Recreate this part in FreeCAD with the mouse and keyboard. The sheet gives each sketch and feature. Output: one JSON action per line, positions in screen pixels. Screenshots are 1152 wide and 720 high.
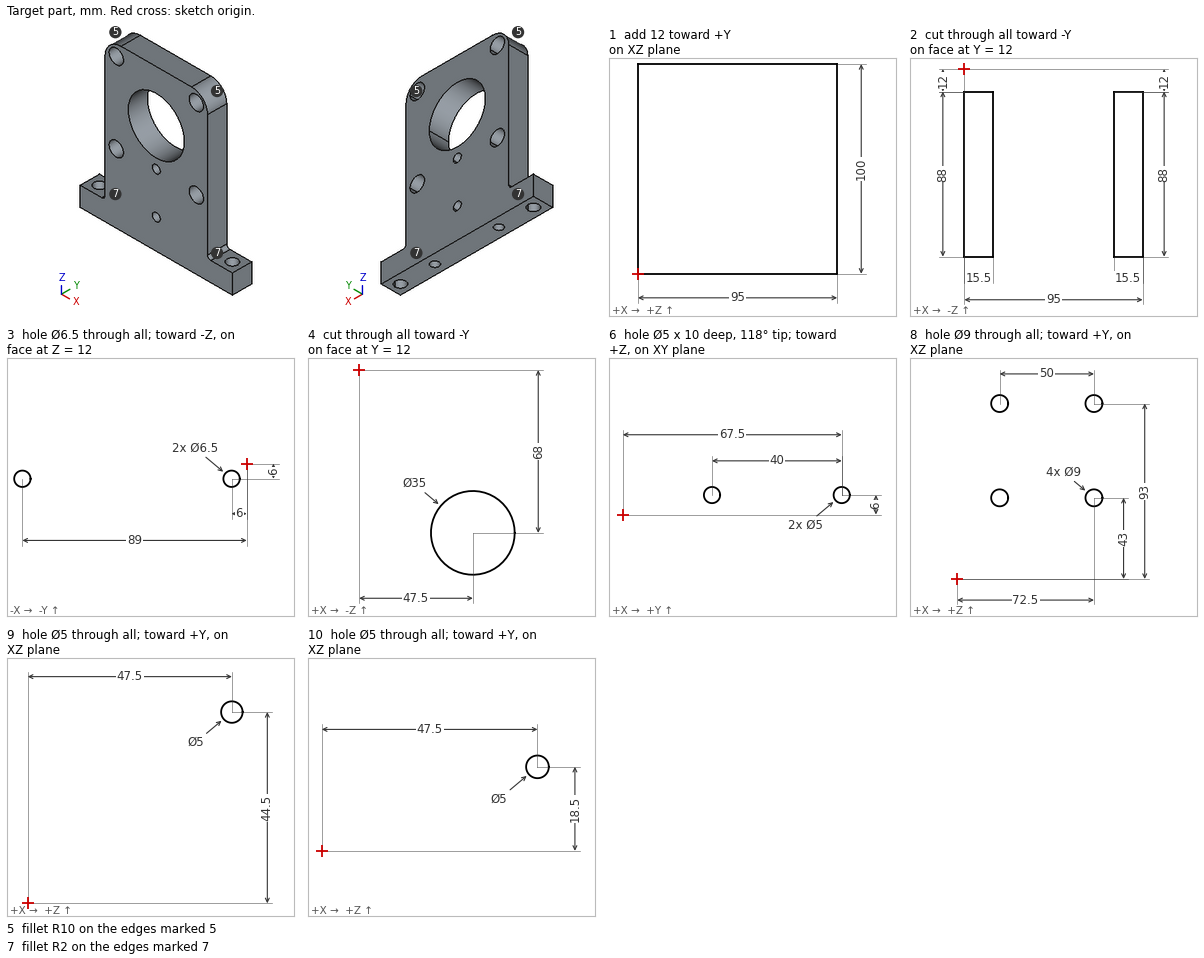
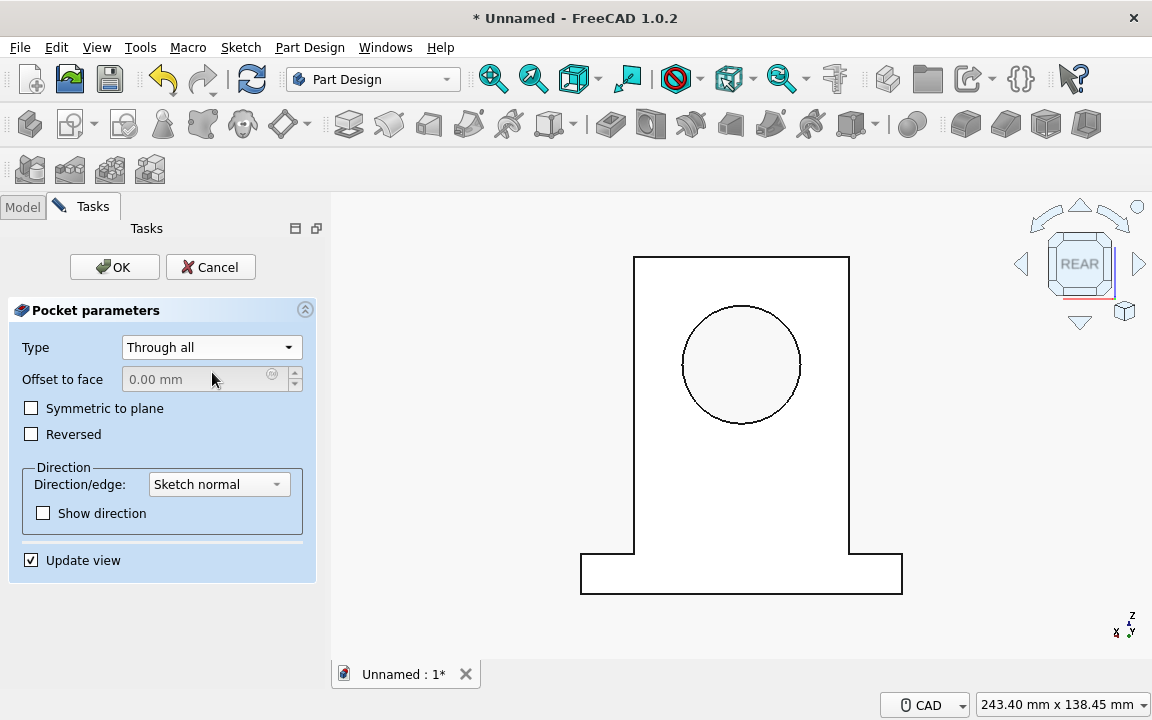
{"action": "left_click", "coordinate": [115, 267]}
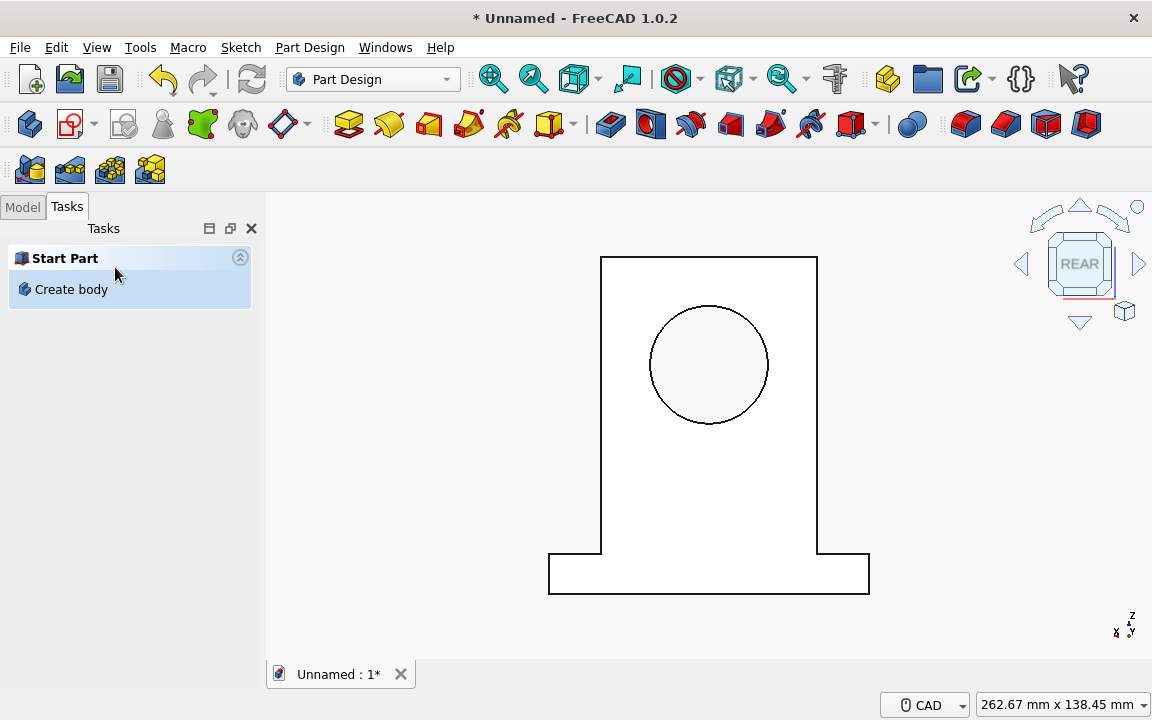
{"action": "key", "text": "0"}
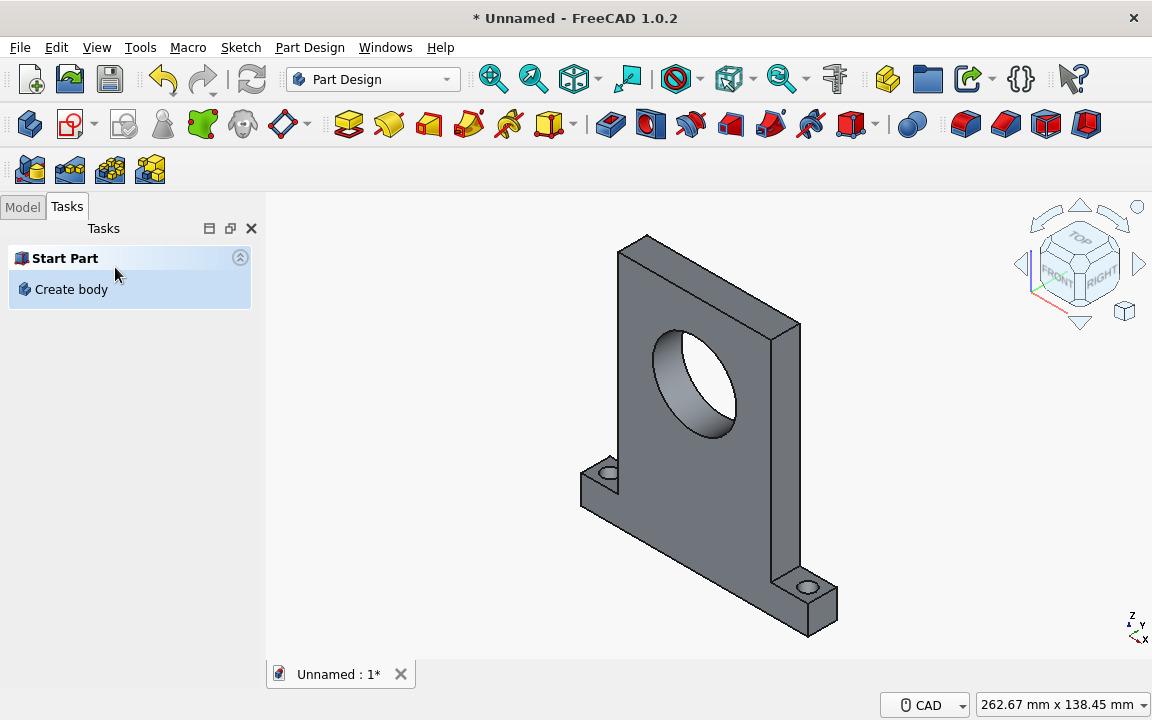
{"action": "left_click", "coordinate": [785, 331]}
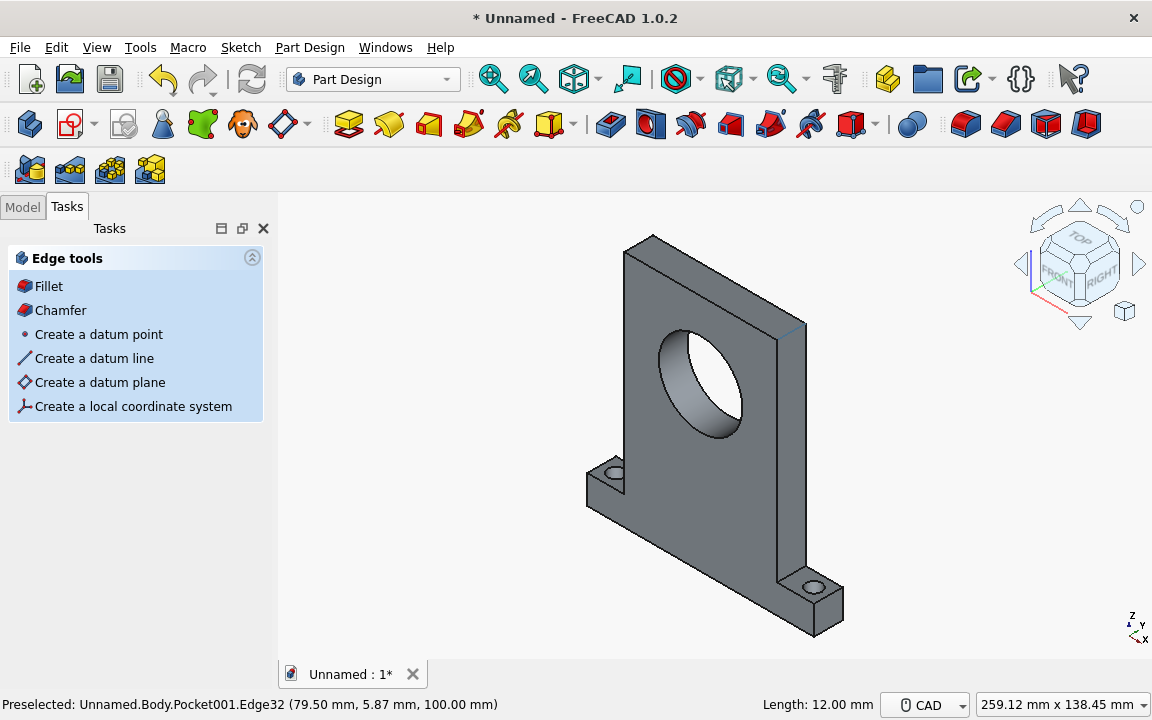
{"action": "key", "text": "2"}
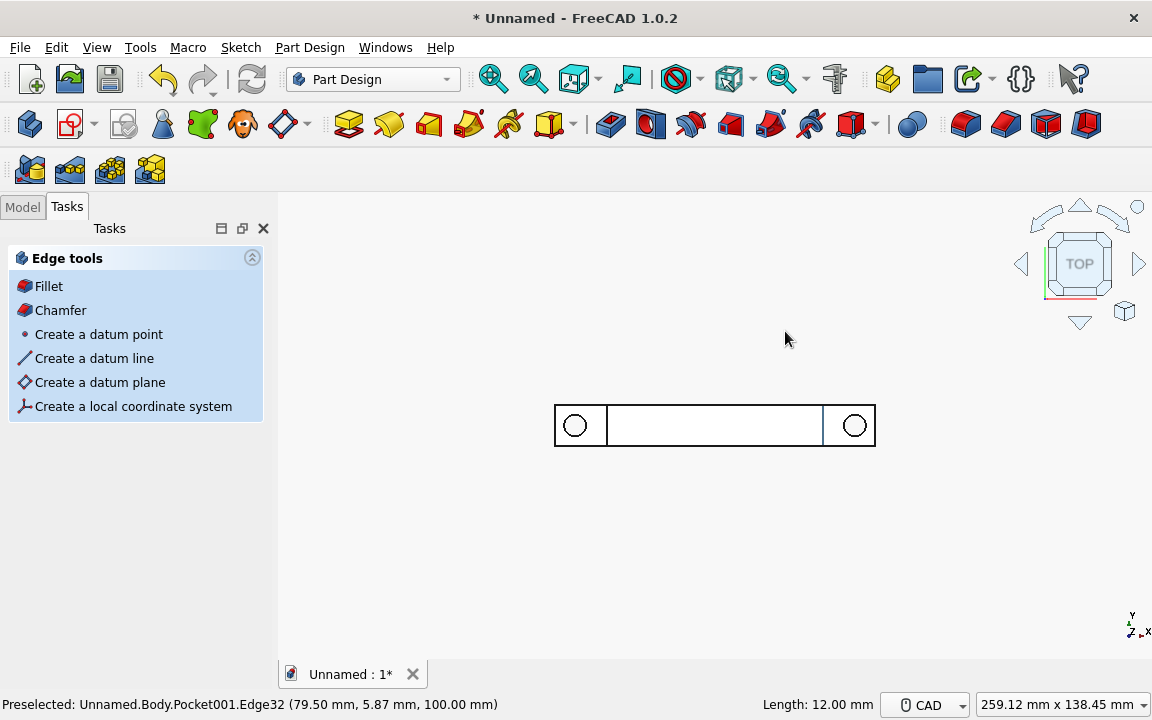
{"action": "left_click", "coordinate": [494, 80]}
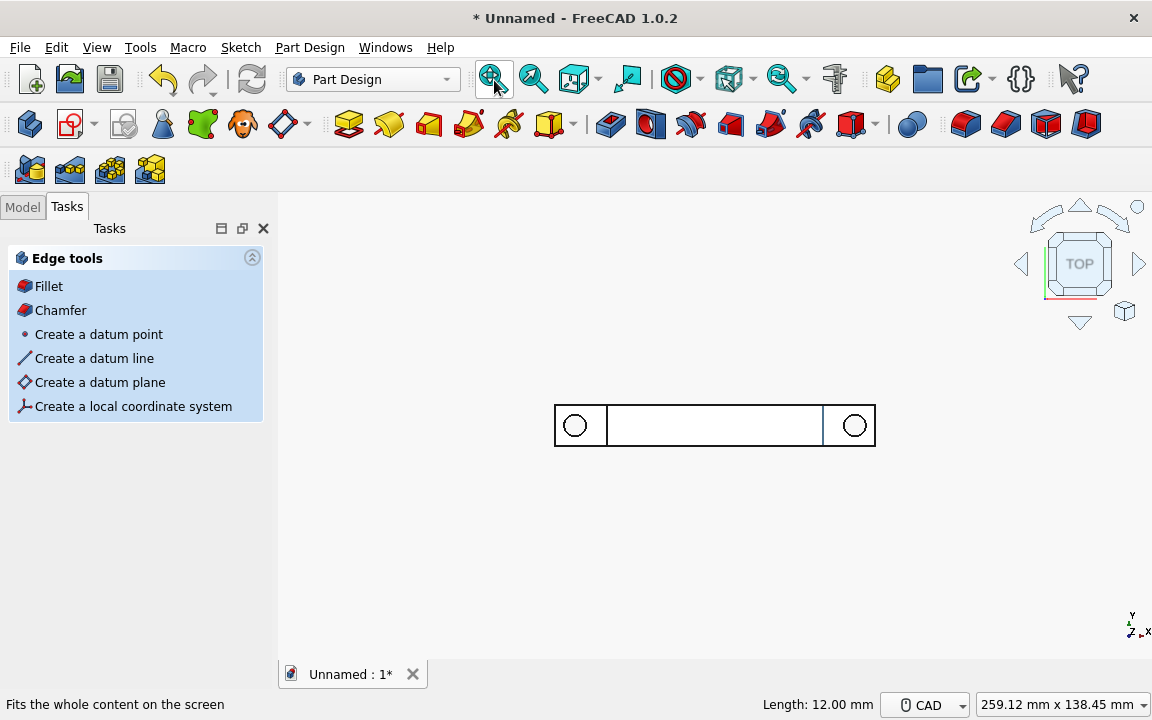
{"action": "left_click", "coordinate": [607, 424], "text": "ctrl"}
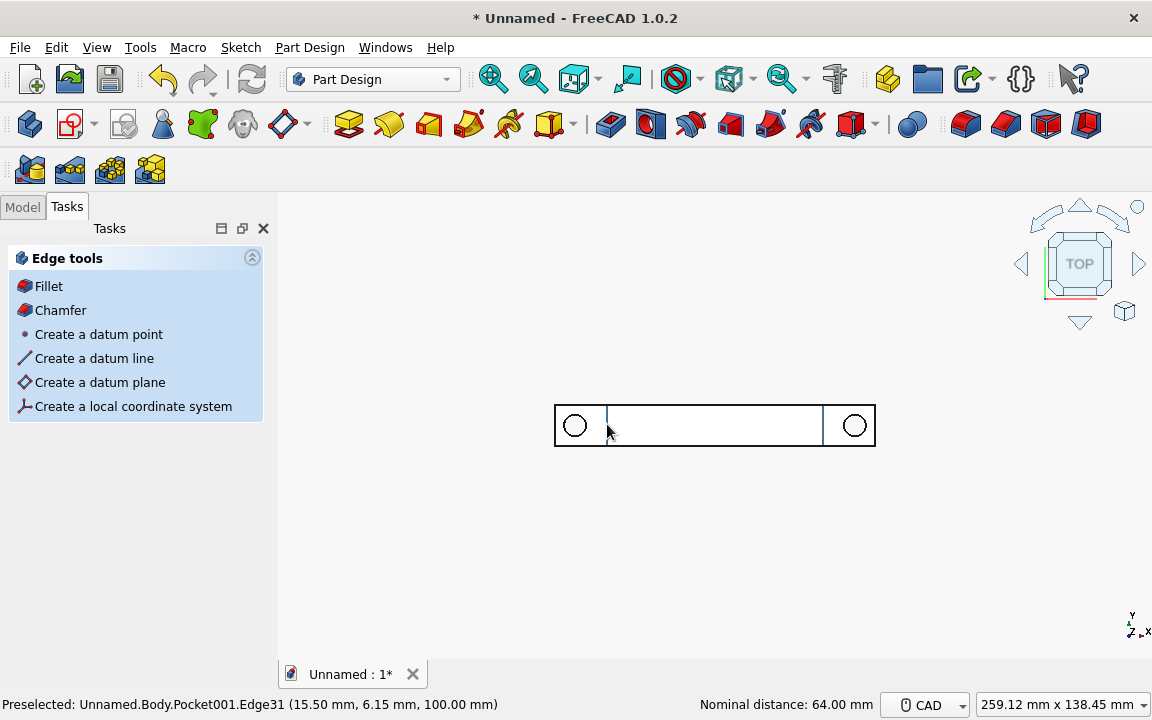
{"action": "left_click", "coordinate": [966, 124]}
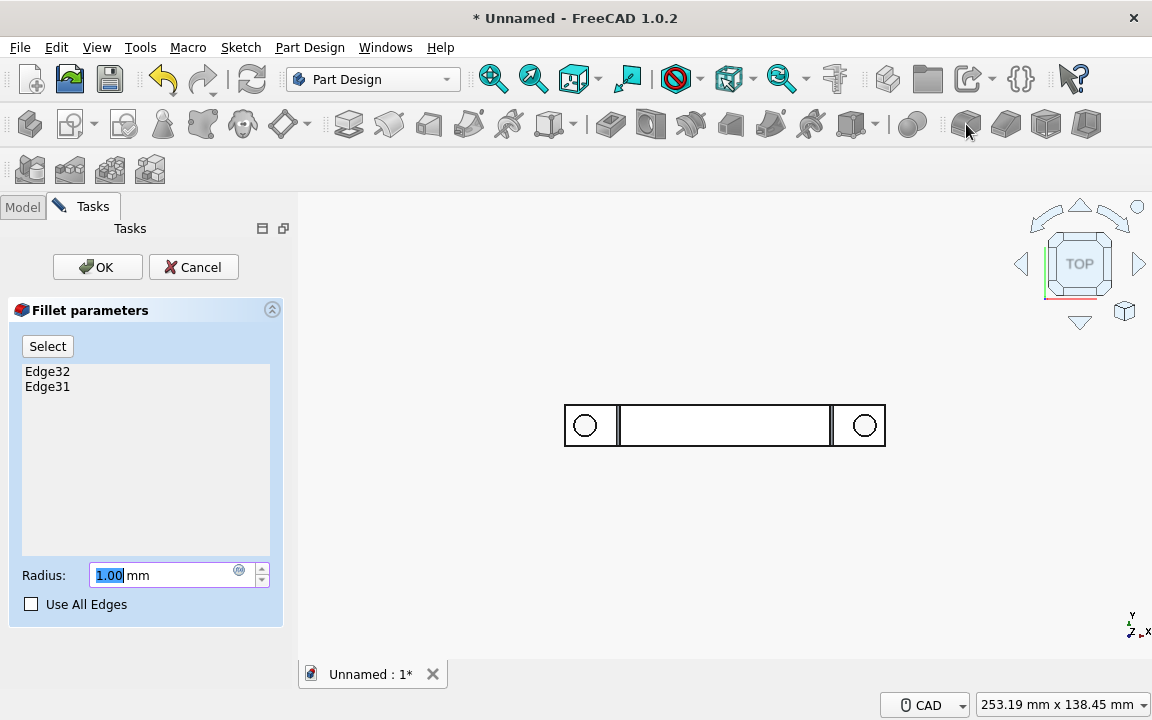
{"action": "type", "text": "10"}
{"action": "key", "text": "Tab"}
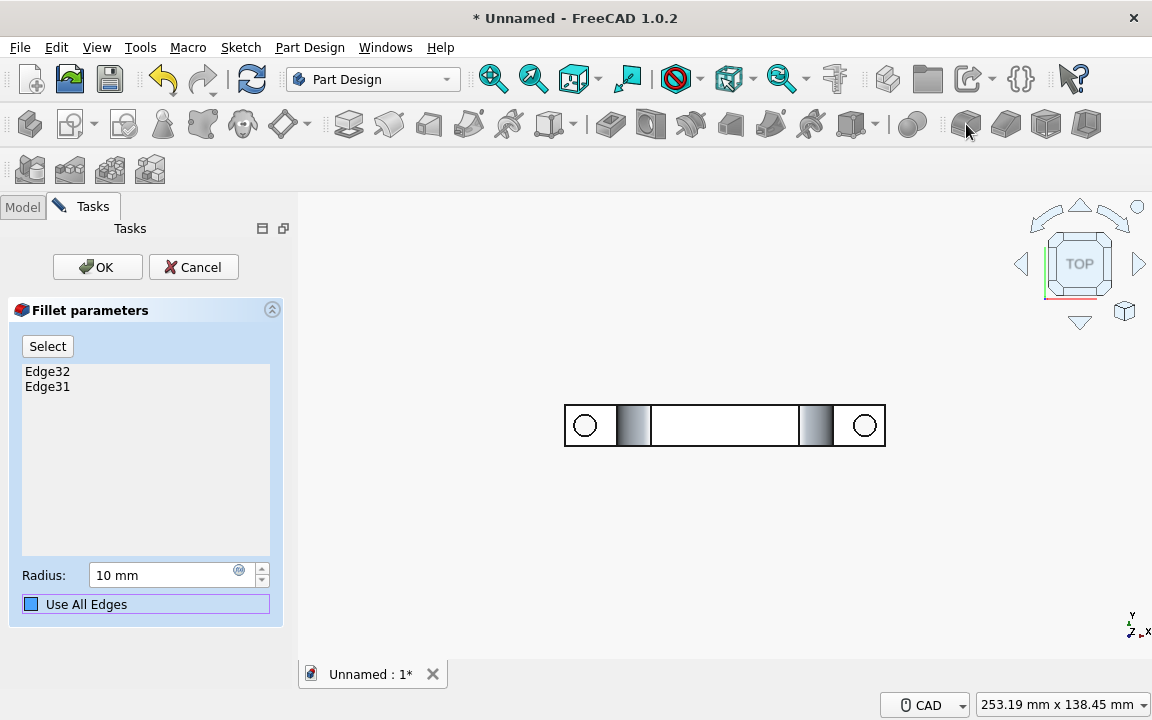
{"action": "left_click", "coordinate": [98, 267]}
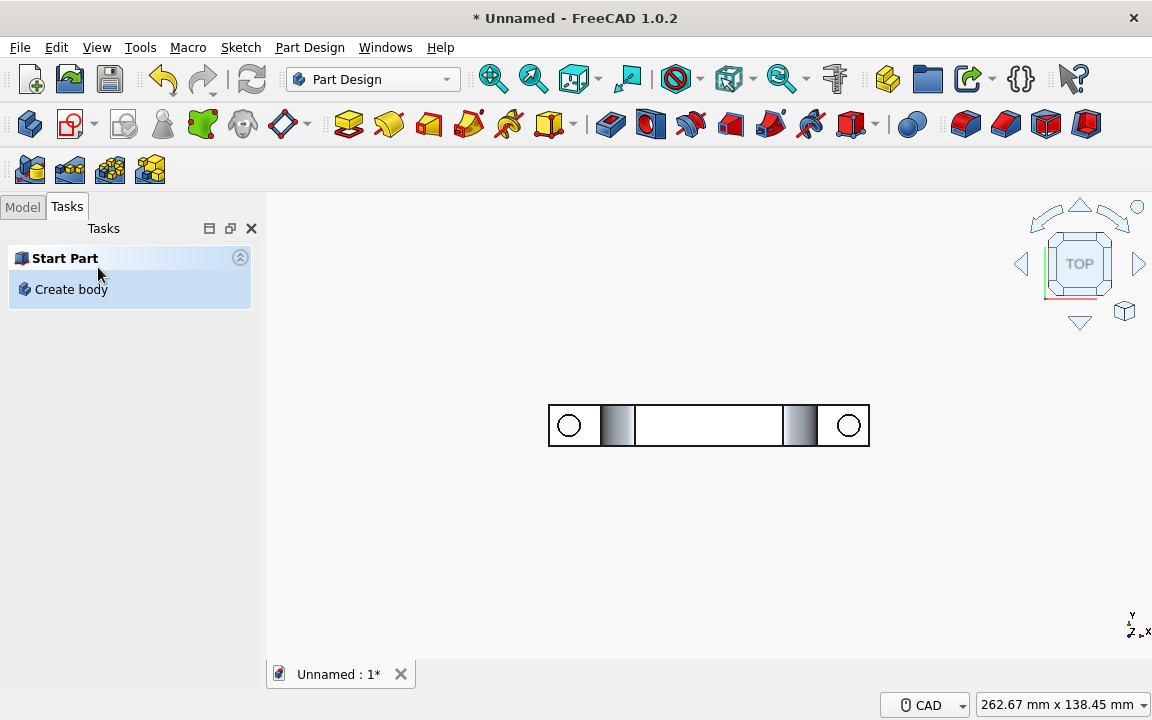
{"action": "left_click", "coordinate": [494, 80]}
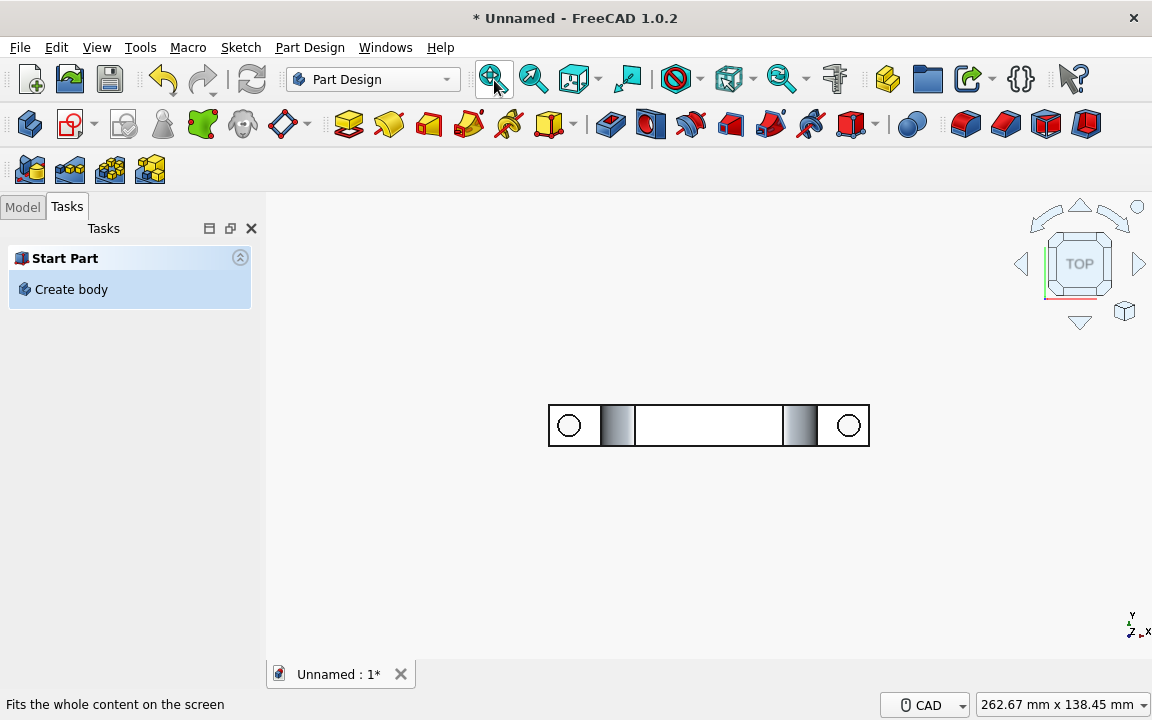
{"action": "left_click", "coordinate": [70, 124]}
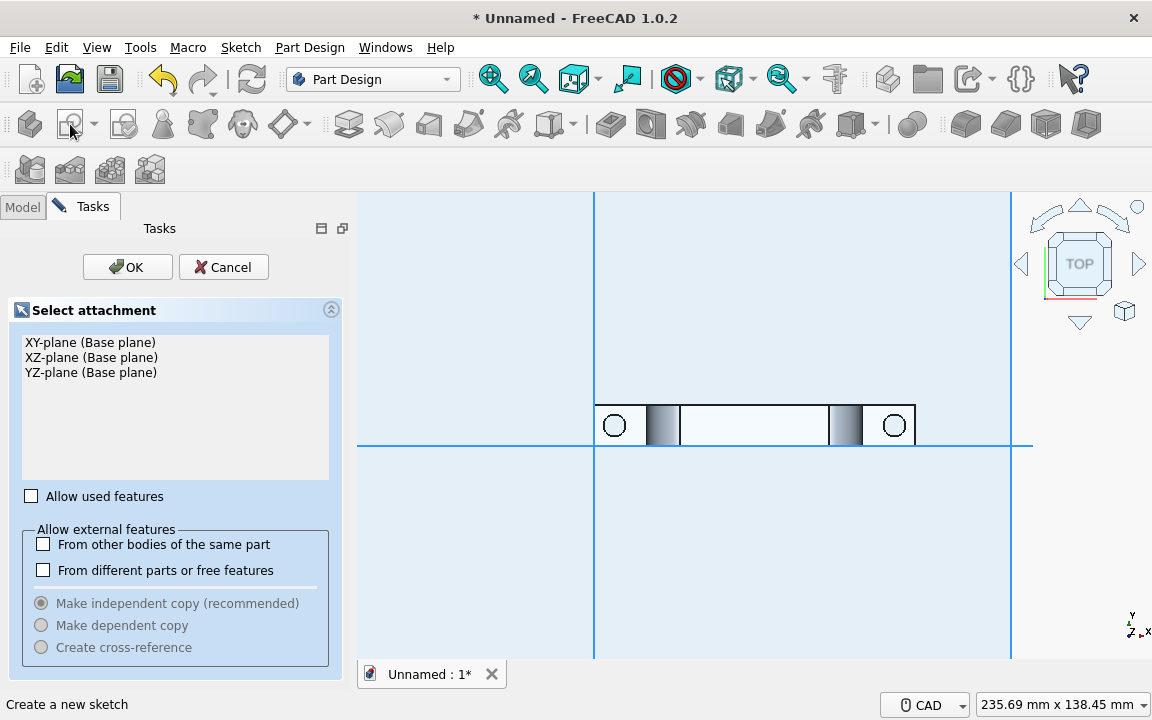
{"action": "left_click", "coordinate": [82, 342]}